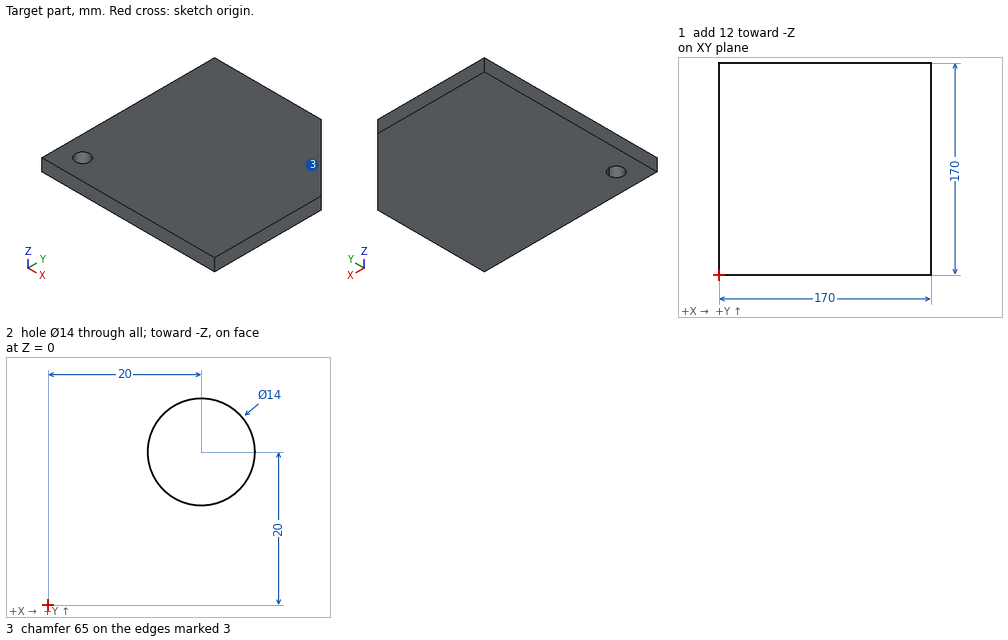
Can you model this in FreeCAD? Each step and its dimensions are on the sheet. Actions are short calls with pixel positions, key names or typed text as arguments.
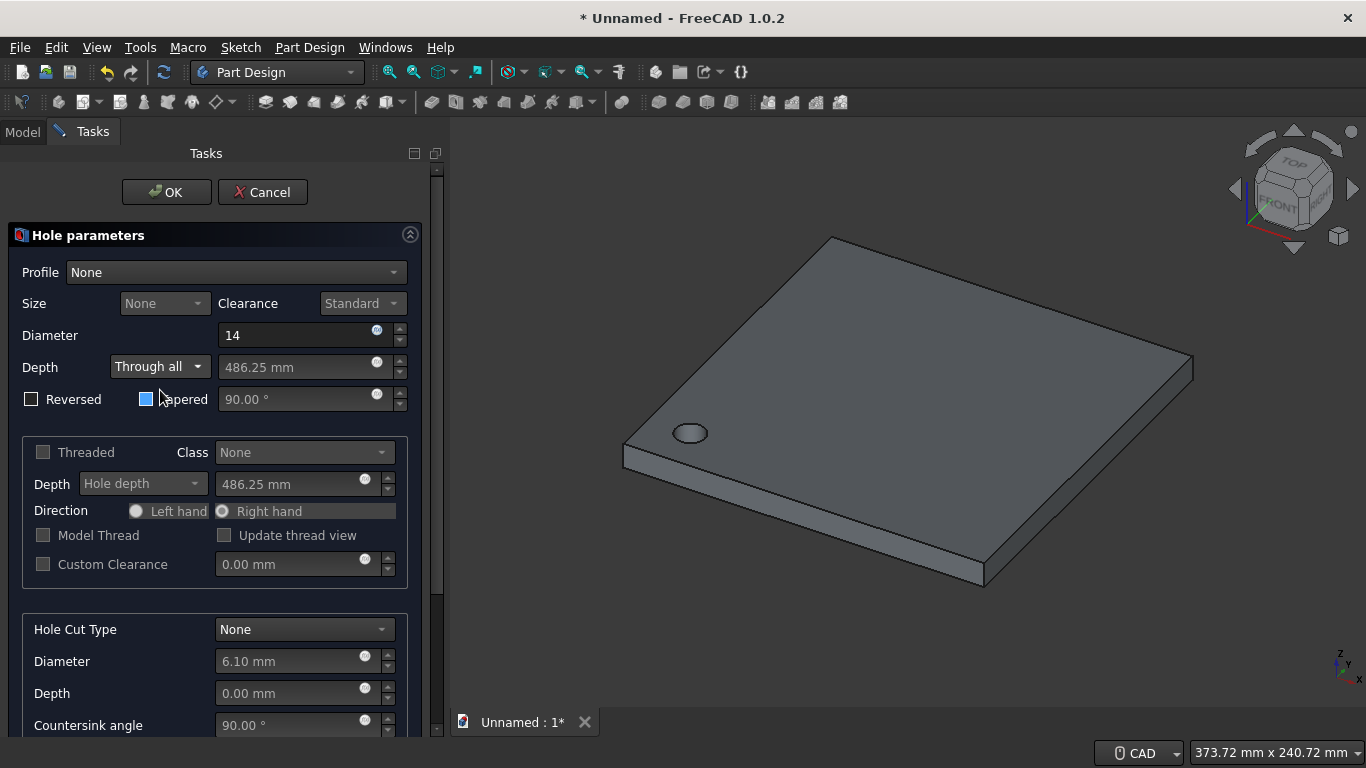
click(167, 192)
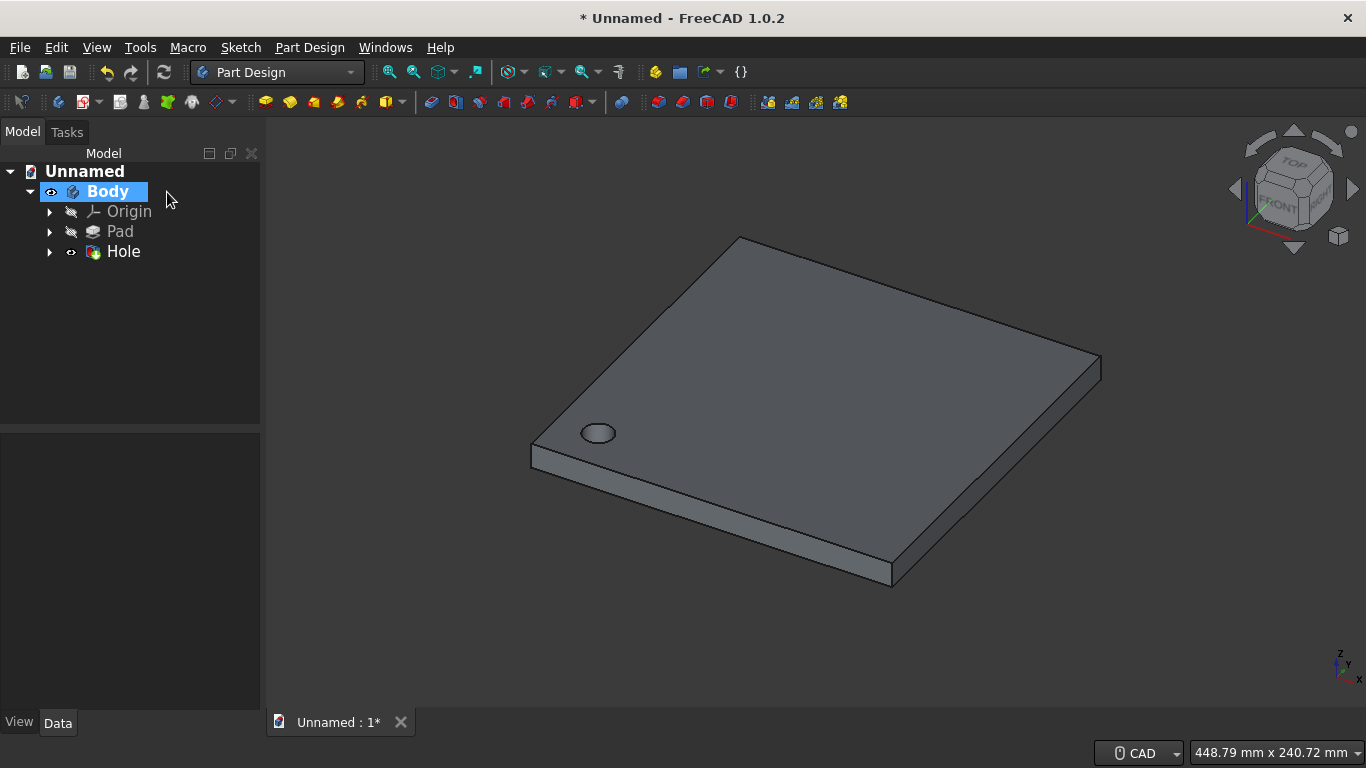
key(0)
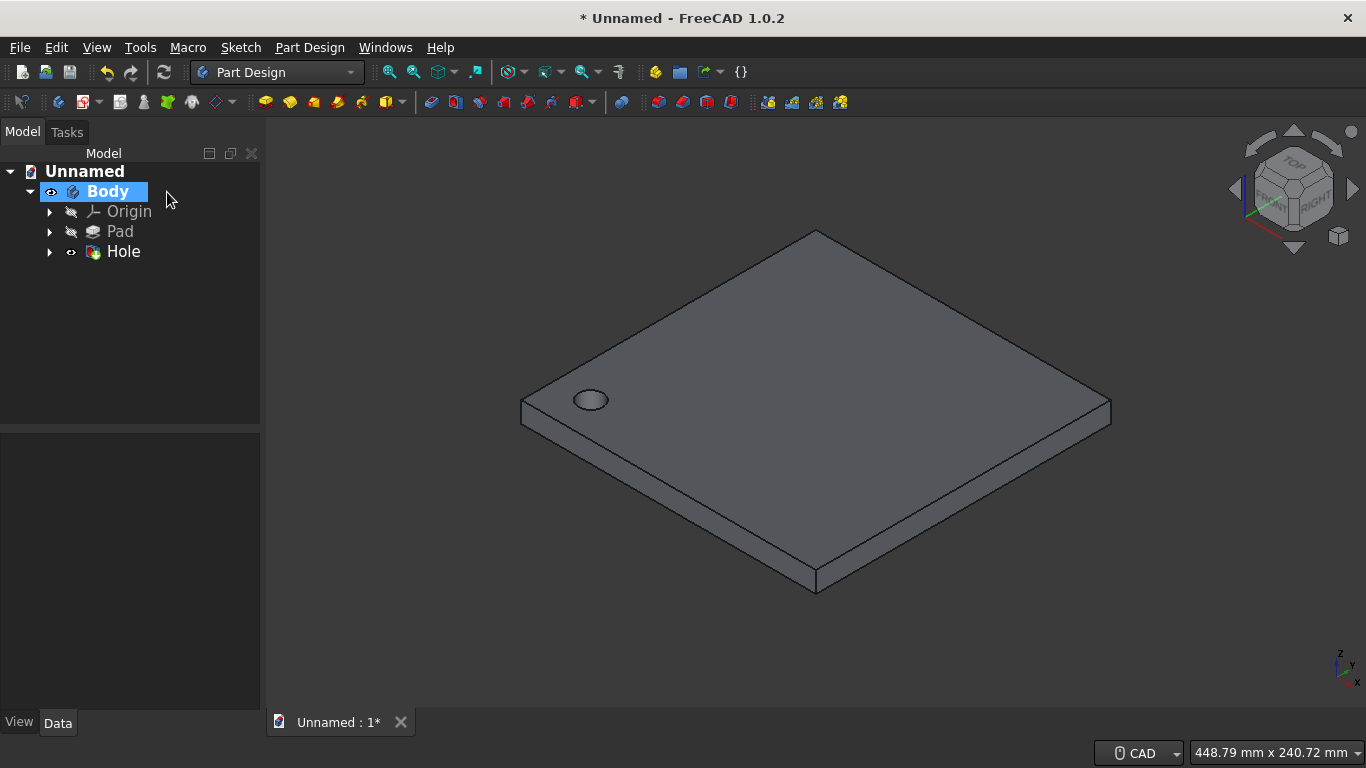
key(2)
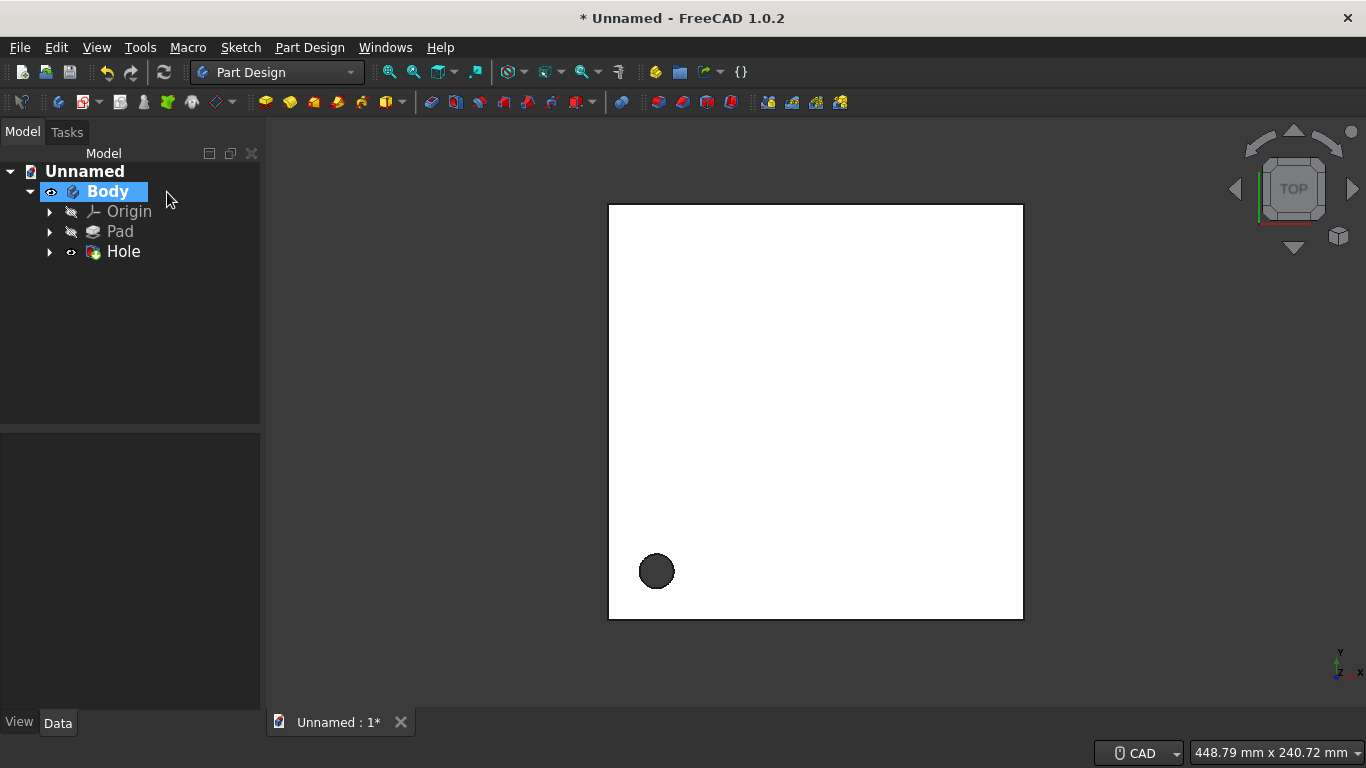
key(1)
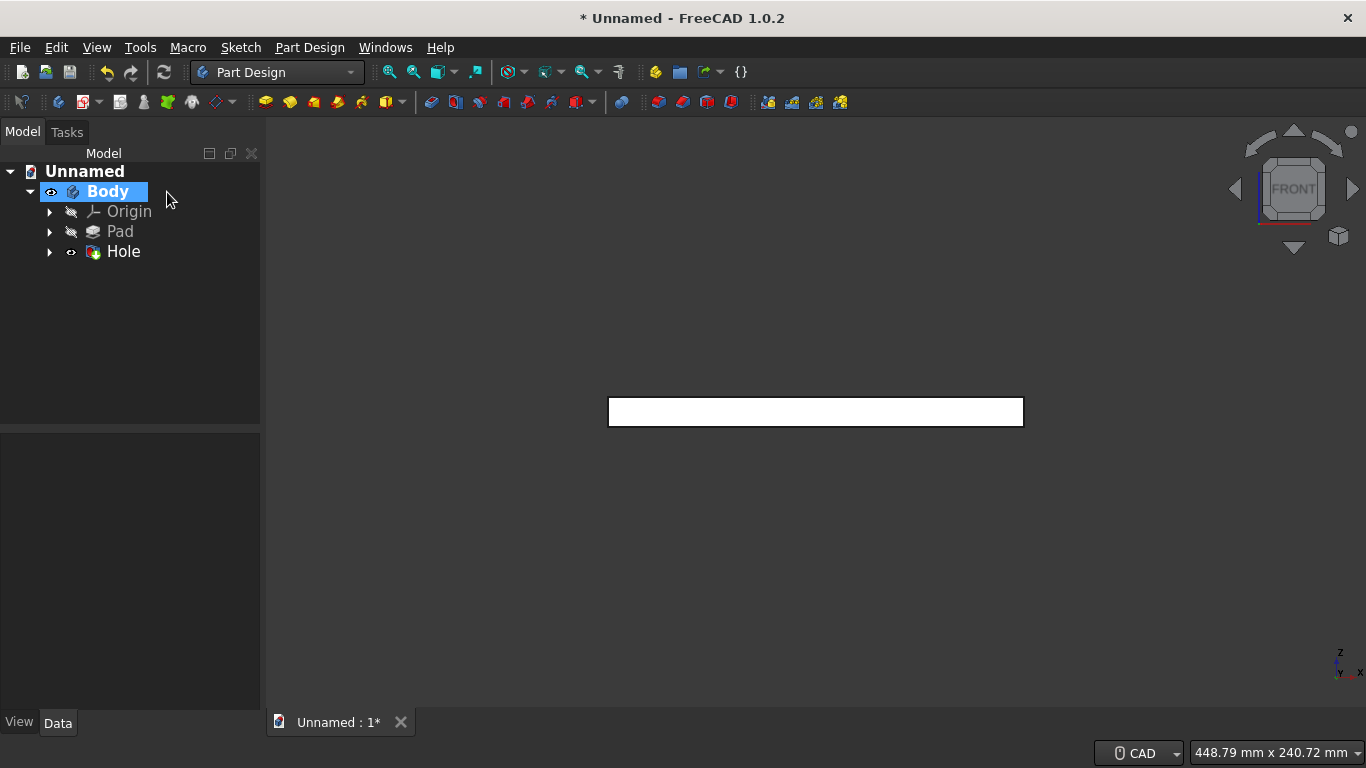
click(390, 72)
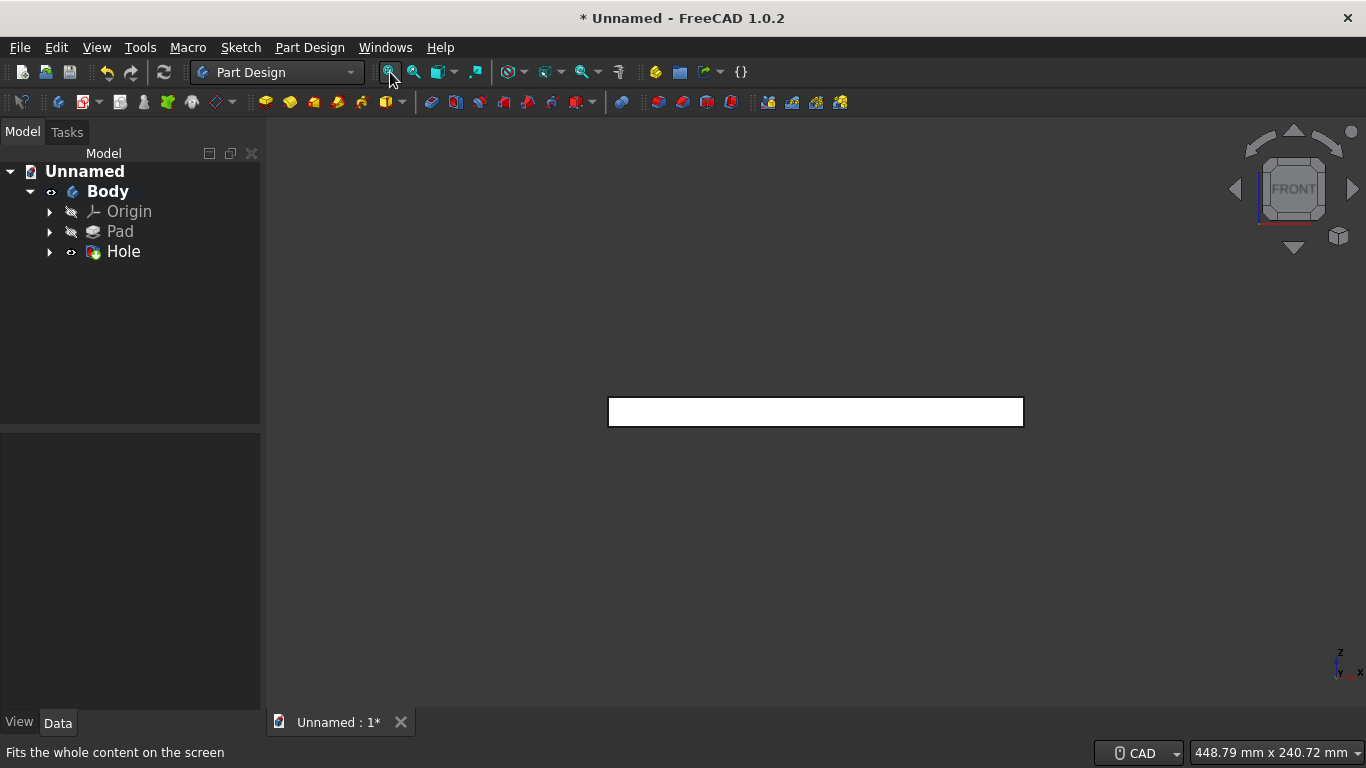
key(3)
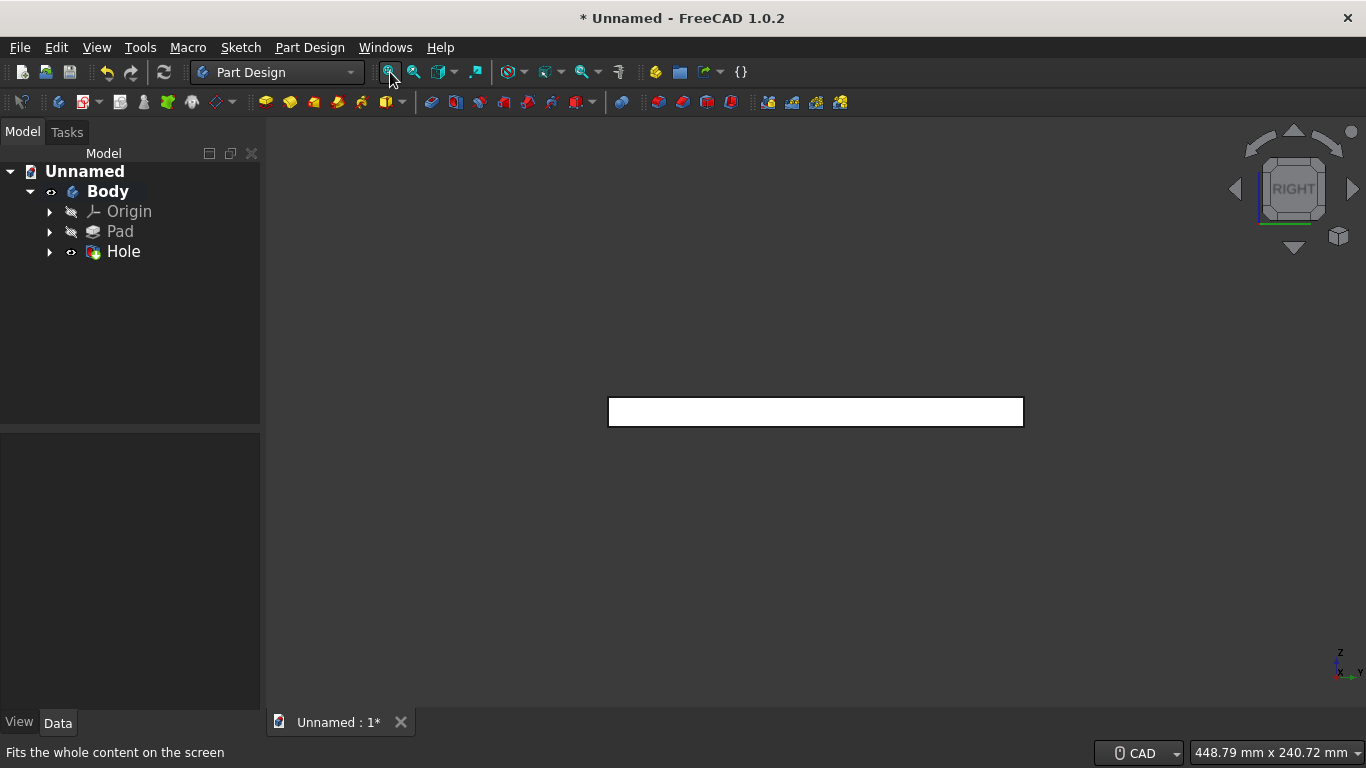
click(390, 72)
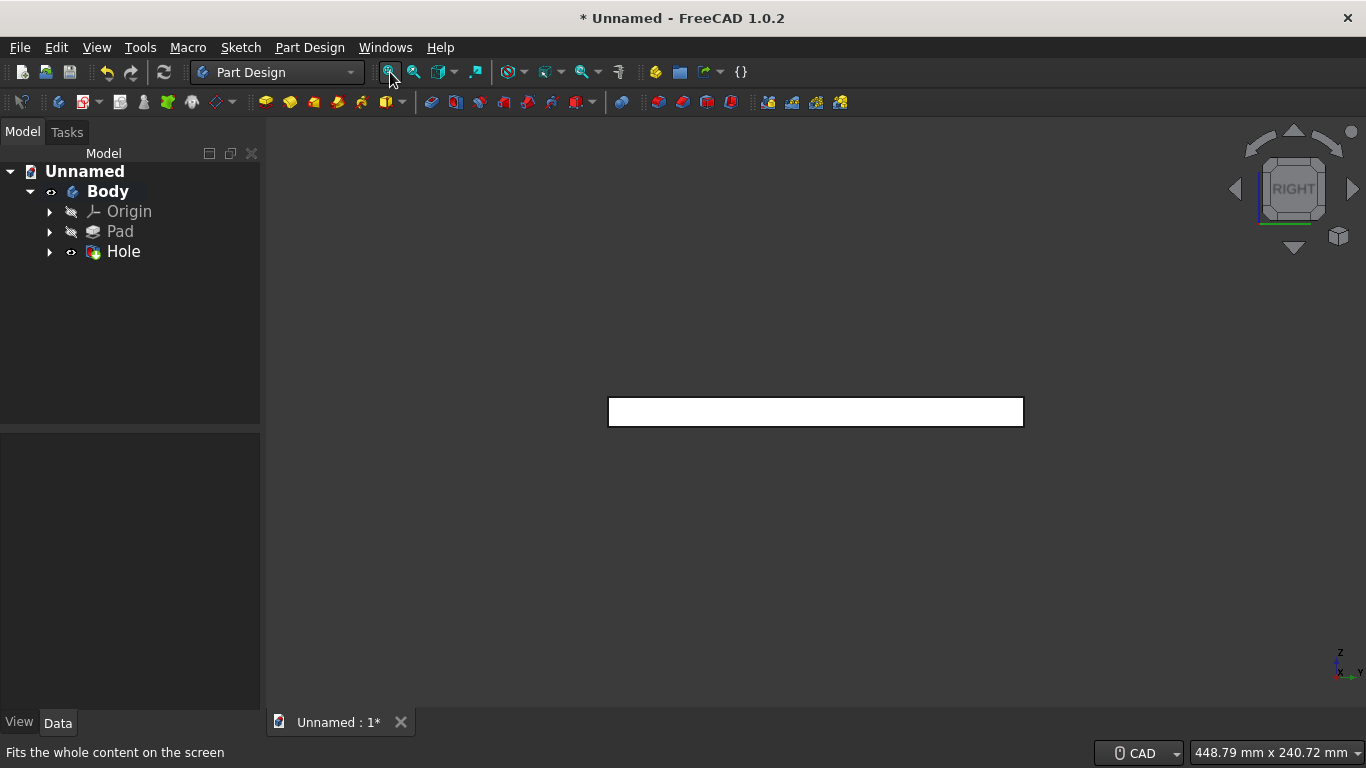
click(1024, 411)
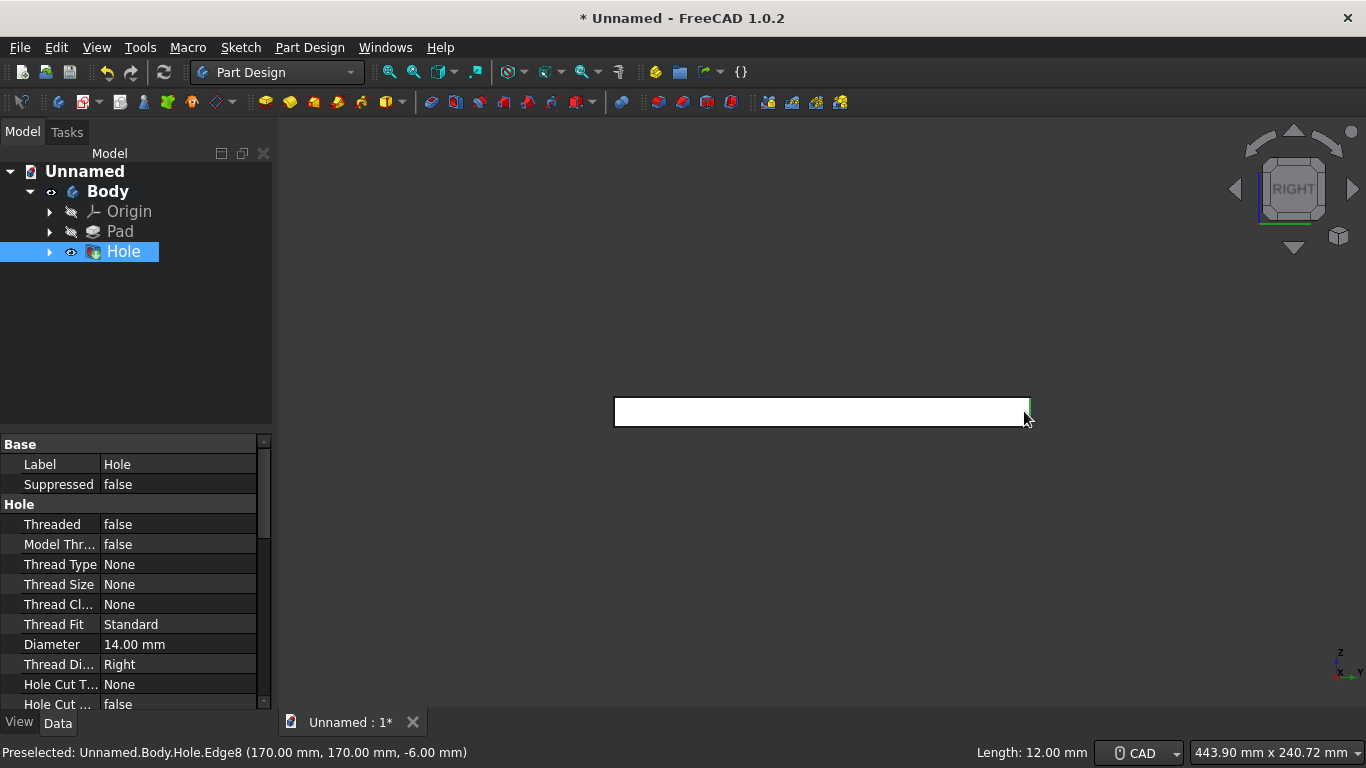
click(684, 102)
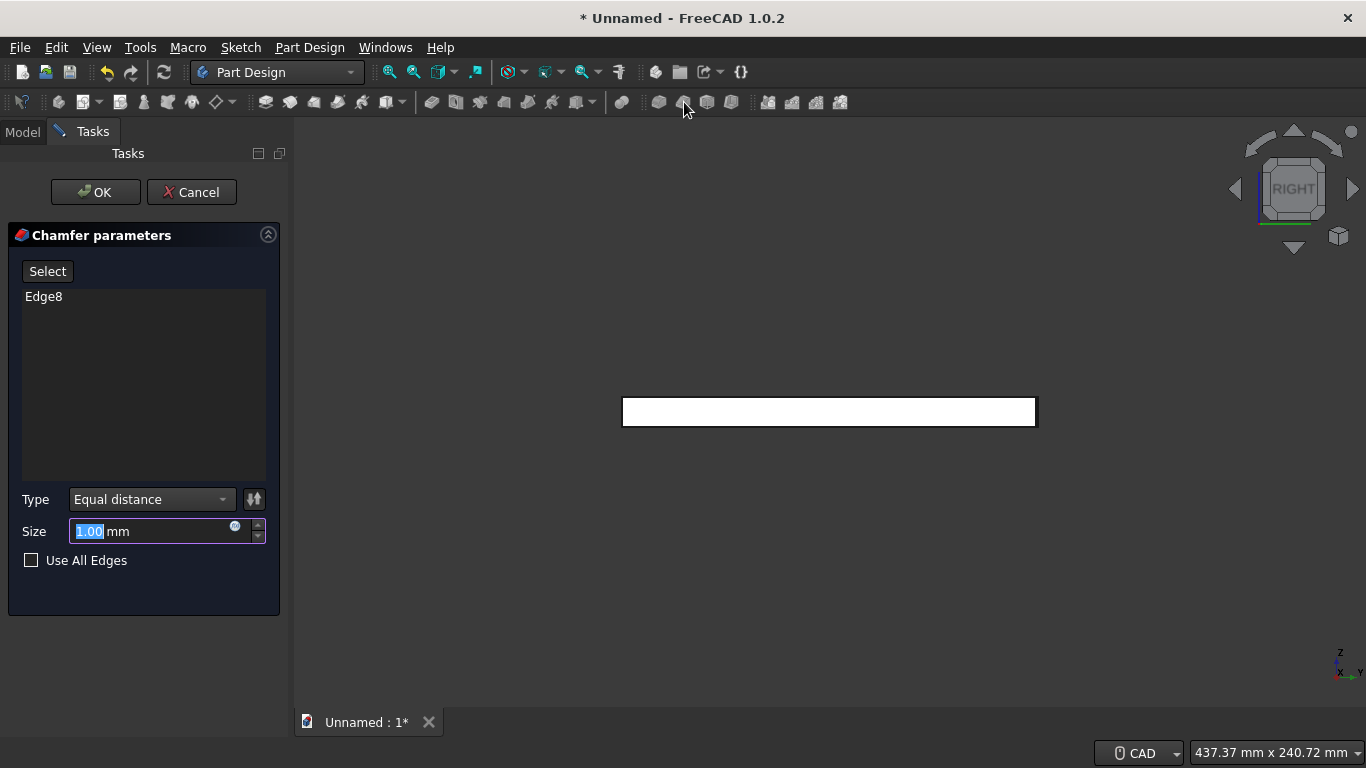
text(65)
key(Tab)